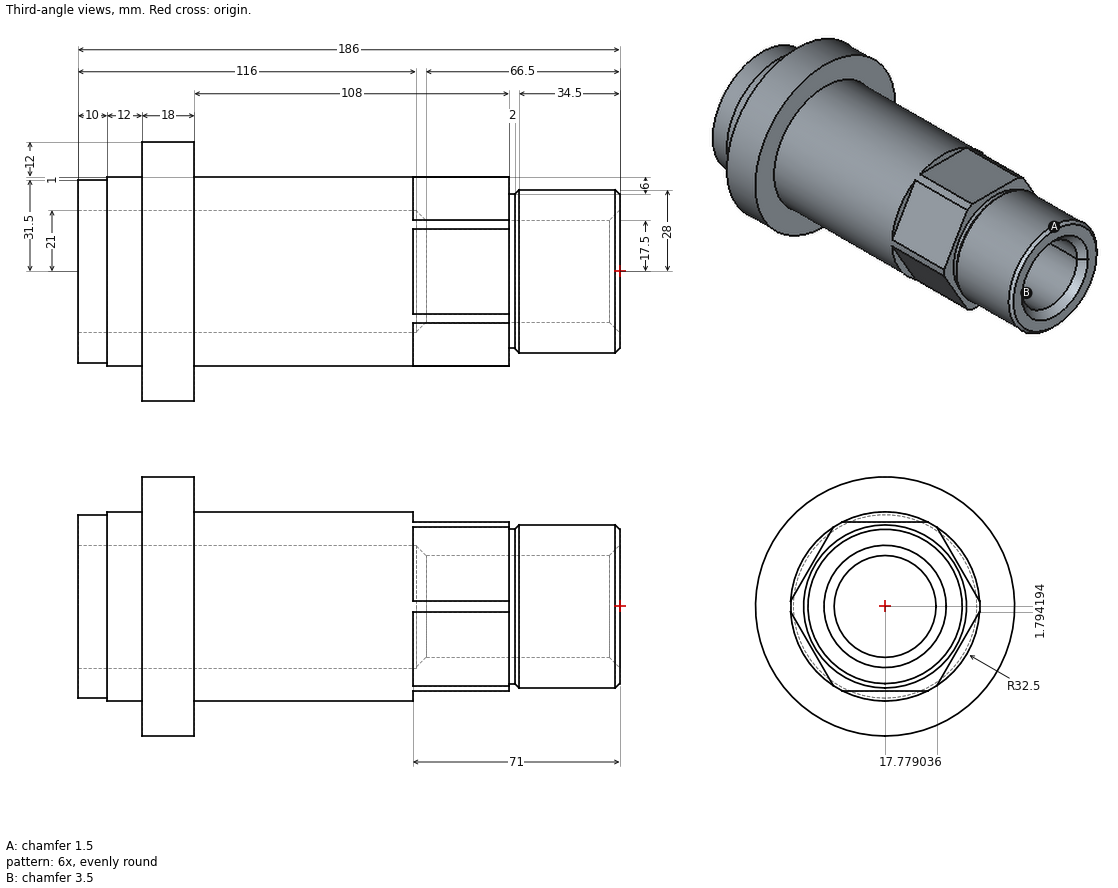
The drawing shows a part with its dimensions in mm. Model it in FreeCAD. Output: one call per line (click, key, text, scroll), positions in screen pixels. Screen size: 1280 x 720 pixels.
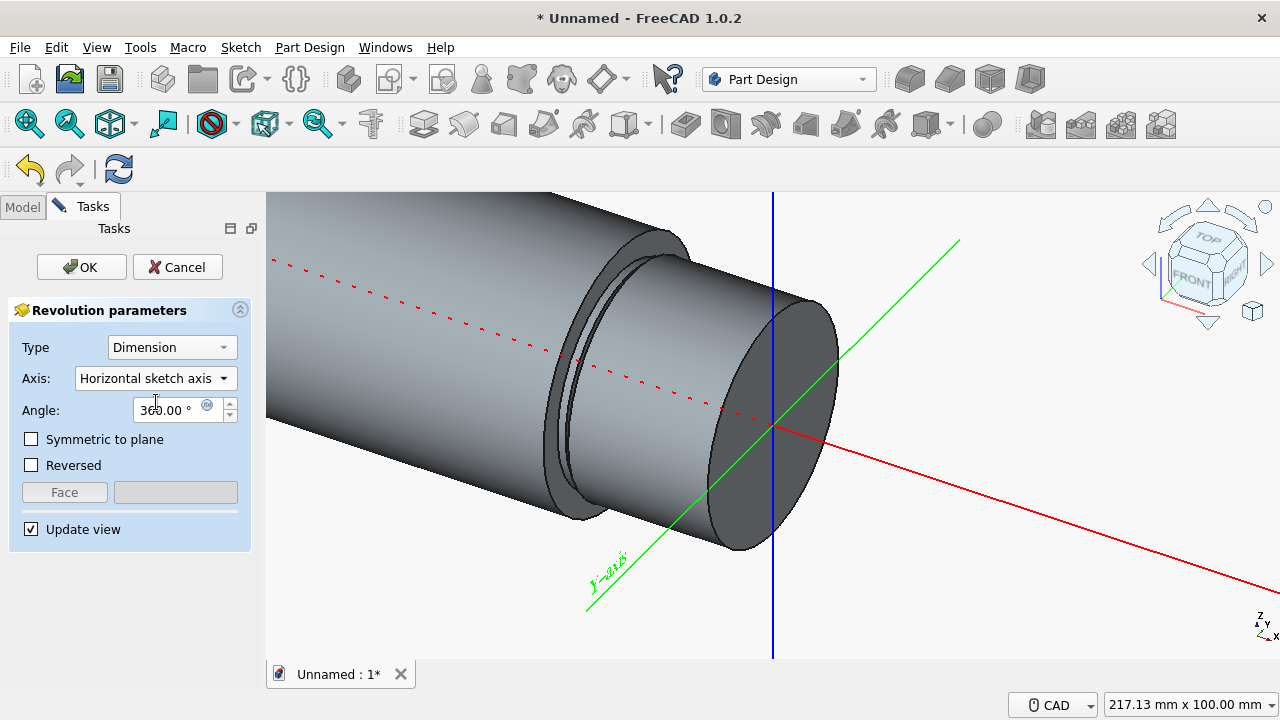
click(82, 267)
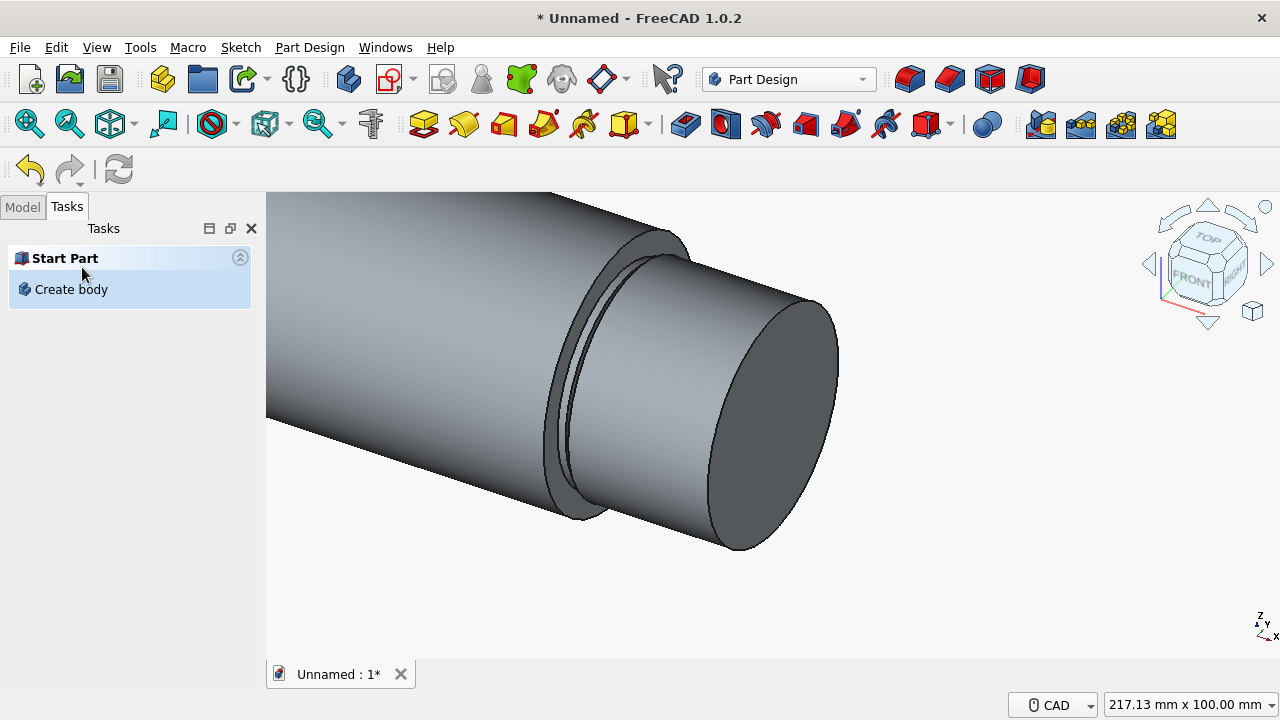
click(30, 124)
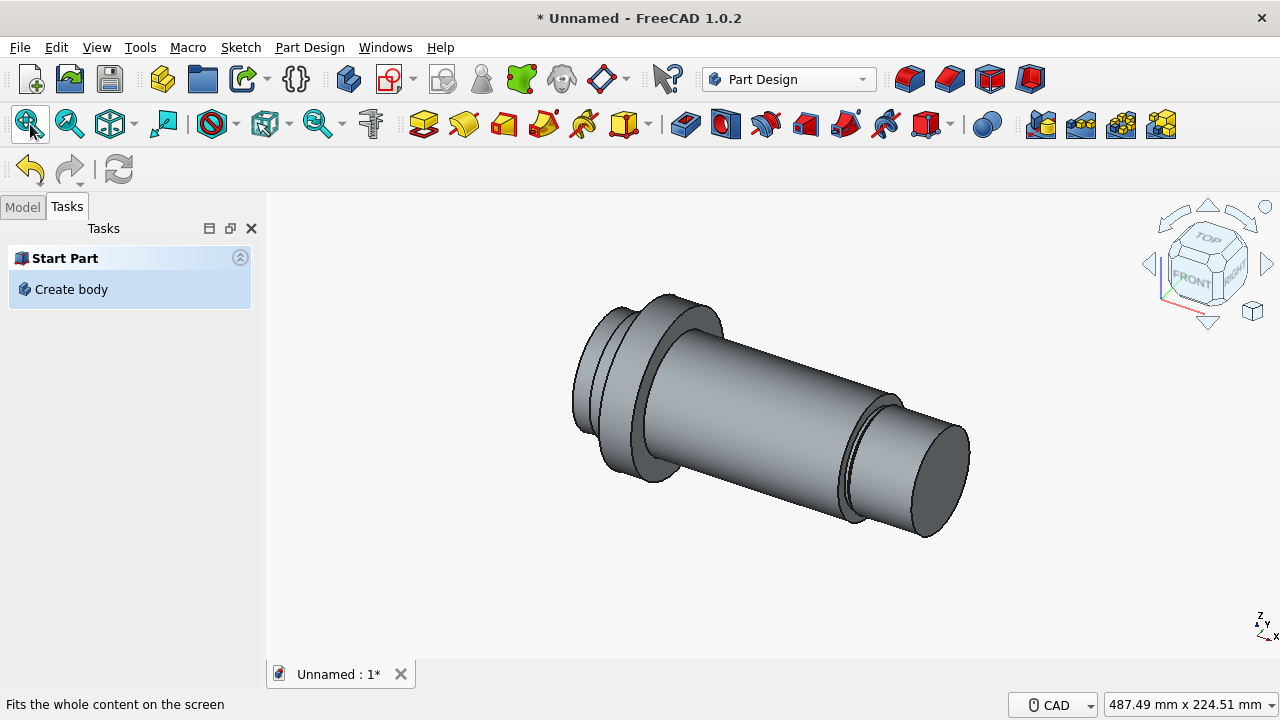
click(911, 509)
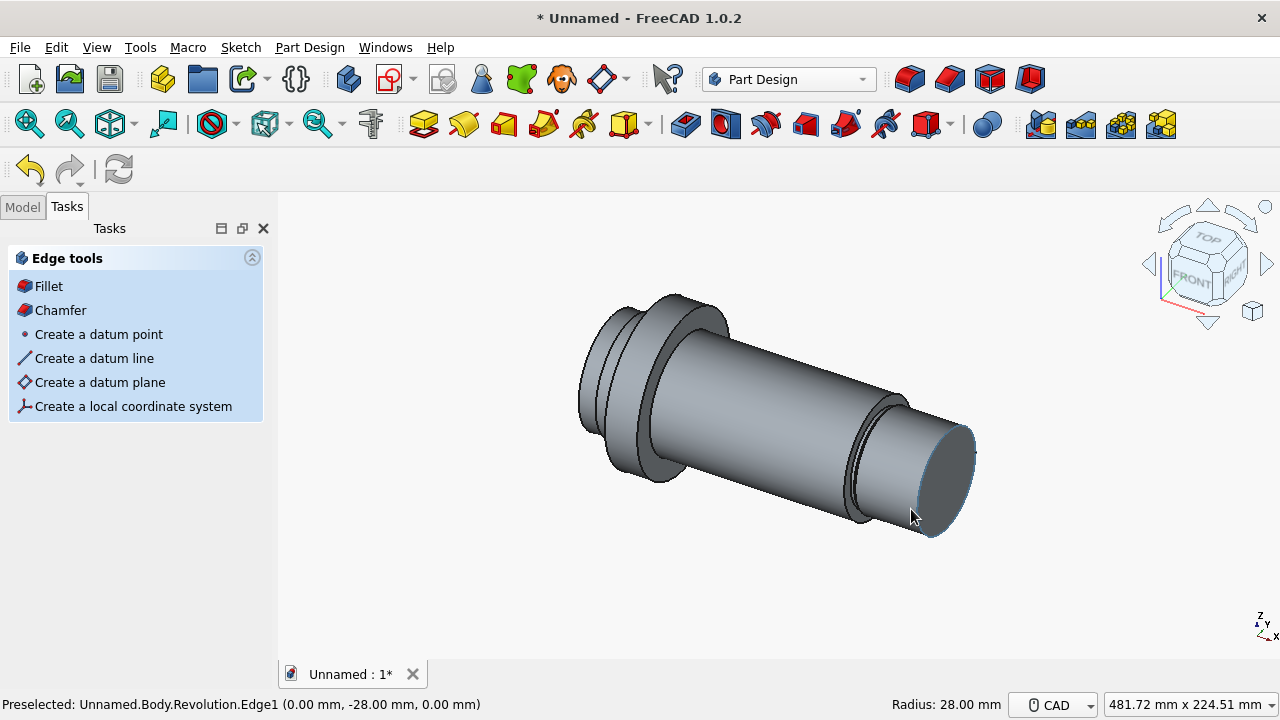
click(950, 80)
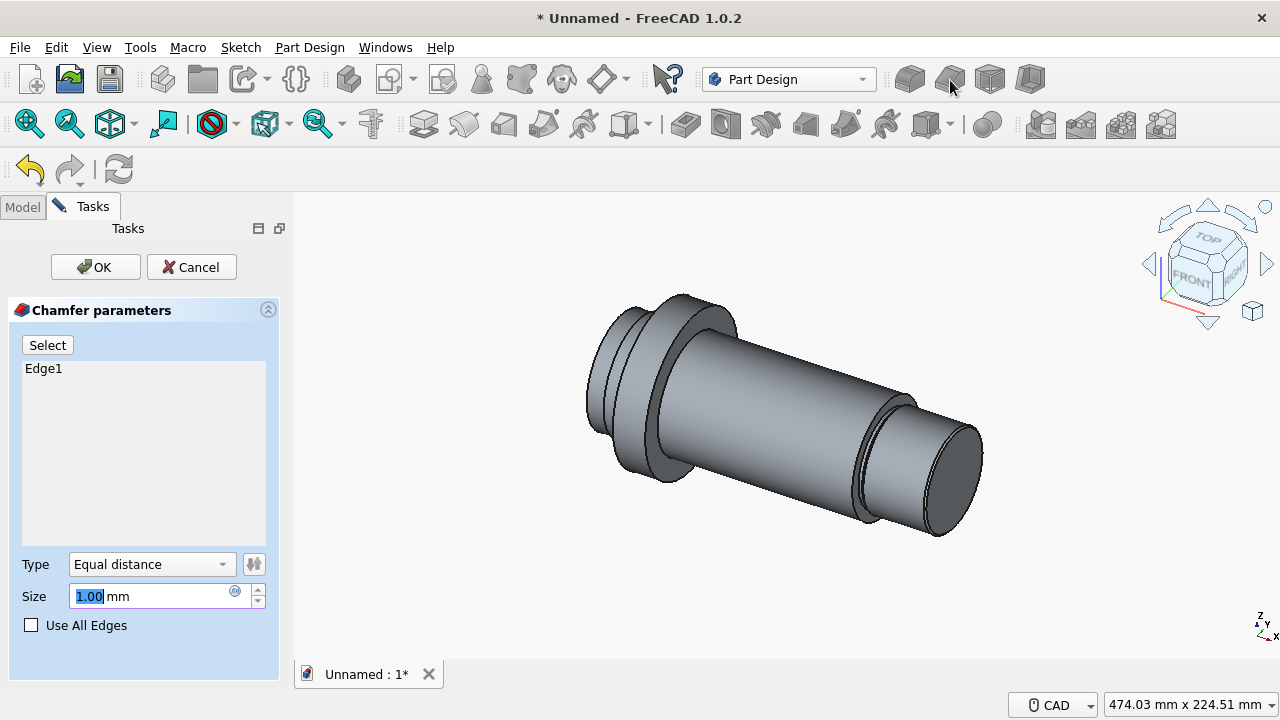
text(1.5)
key(Tab)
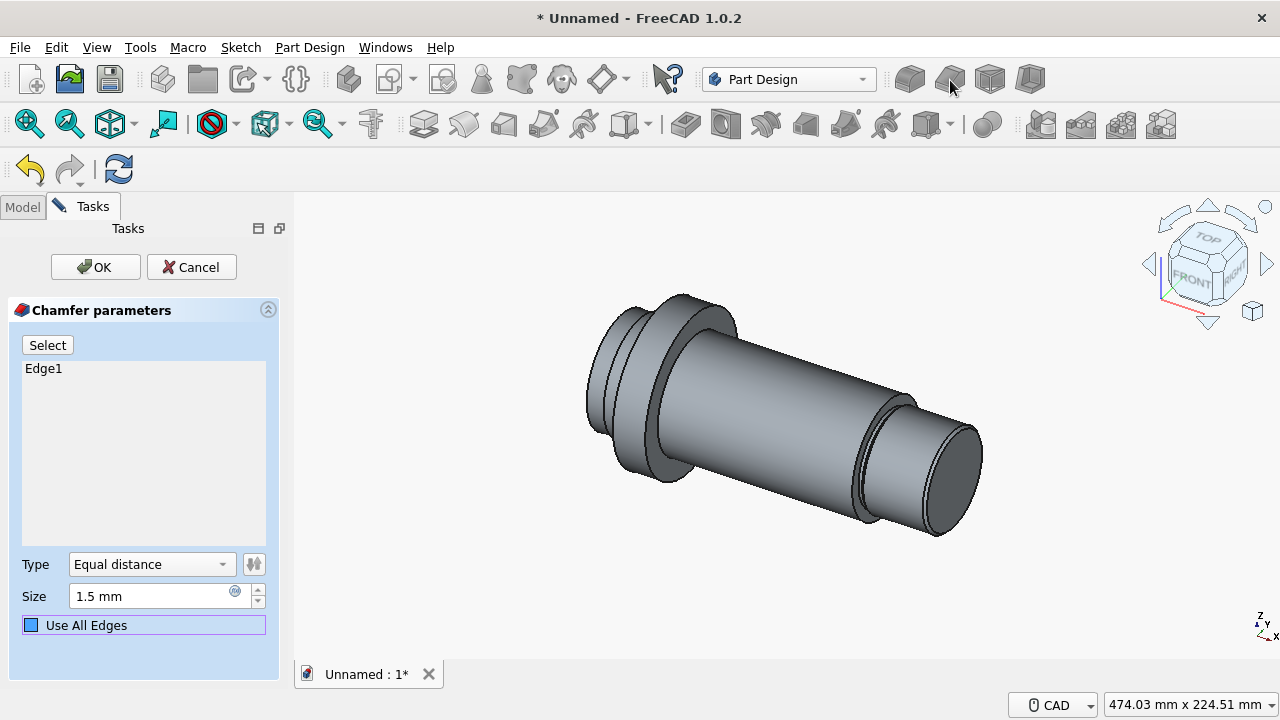
click(96, 267)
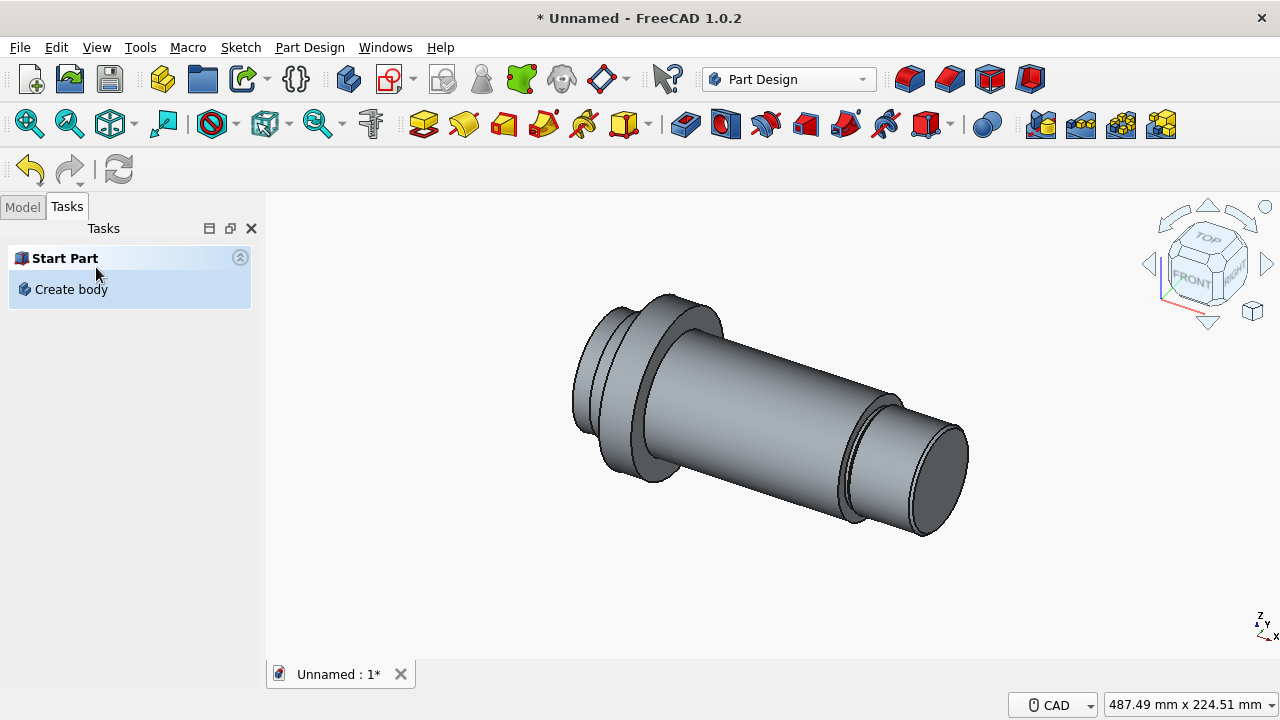
click(23, 206)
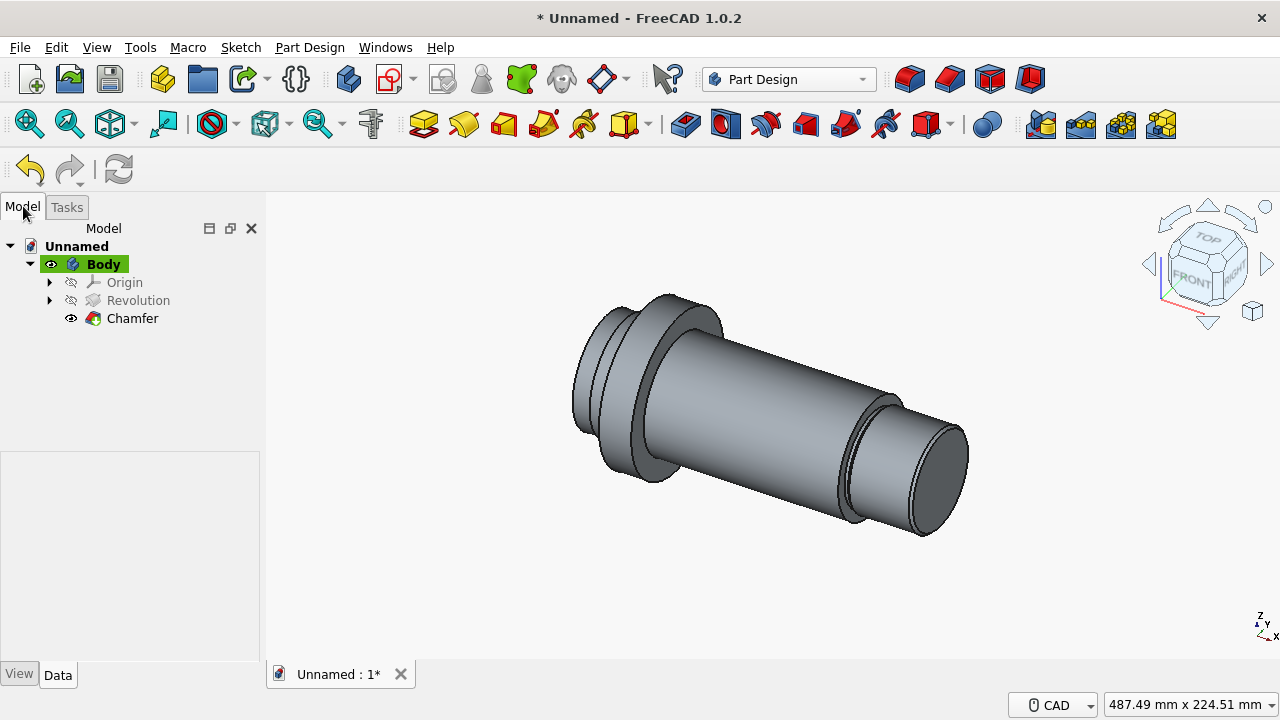
click(50, 282)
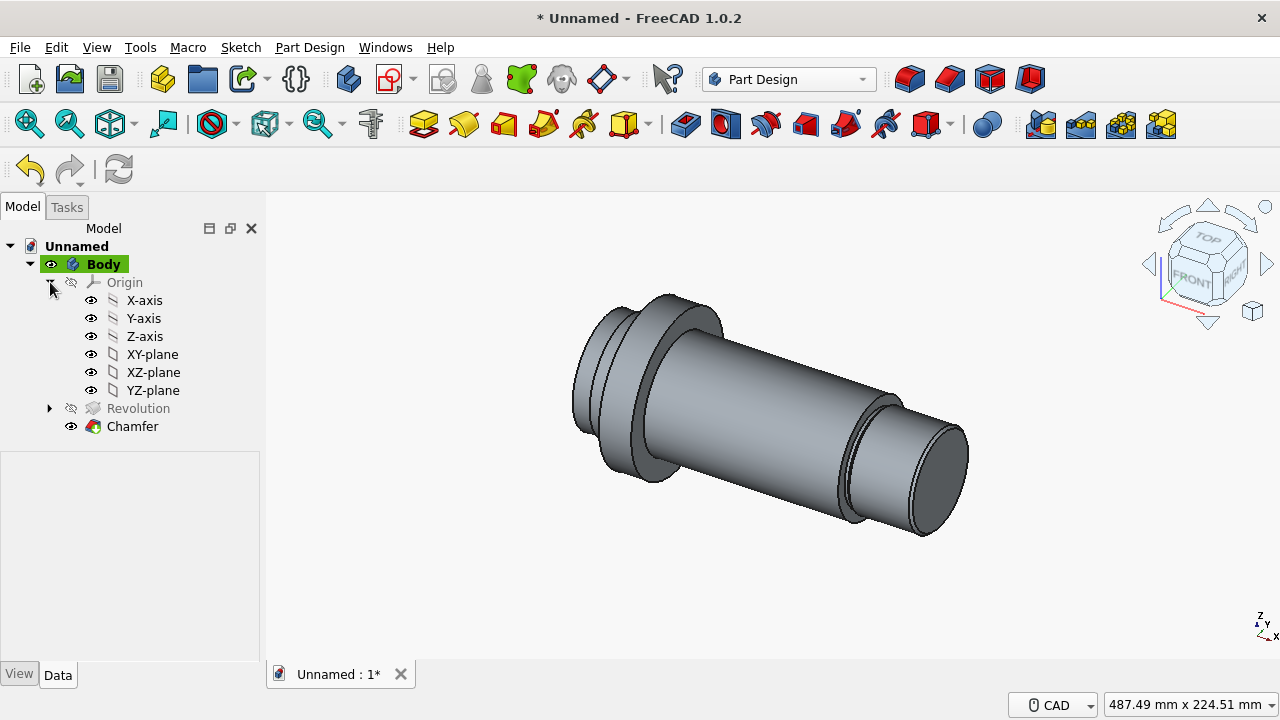
click(136, 390)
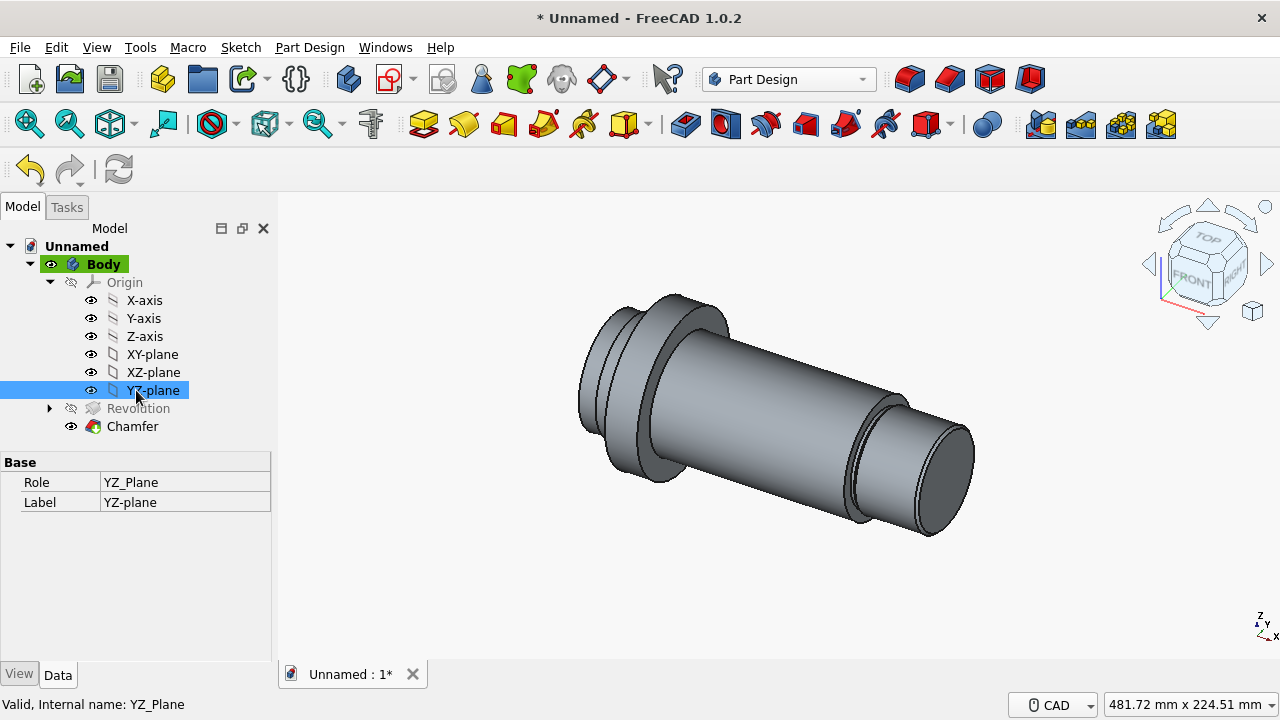
click(602, 80)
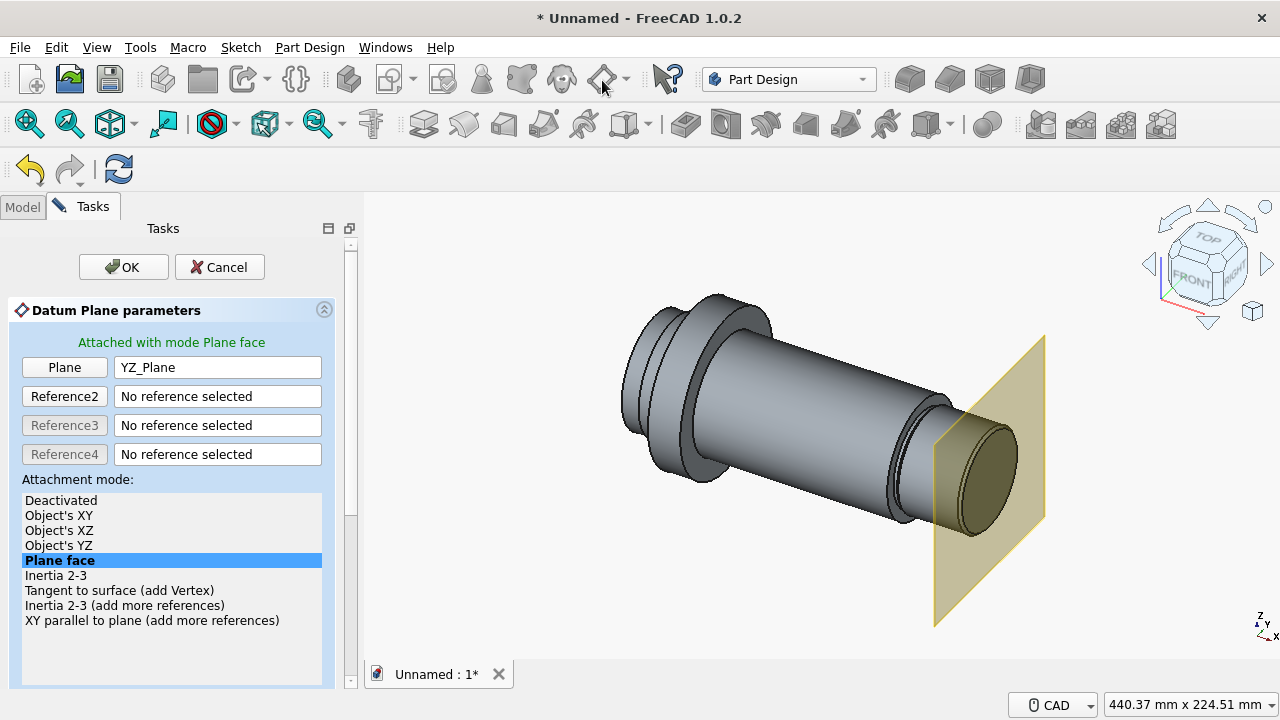
scroll(351, 463, down, 3)